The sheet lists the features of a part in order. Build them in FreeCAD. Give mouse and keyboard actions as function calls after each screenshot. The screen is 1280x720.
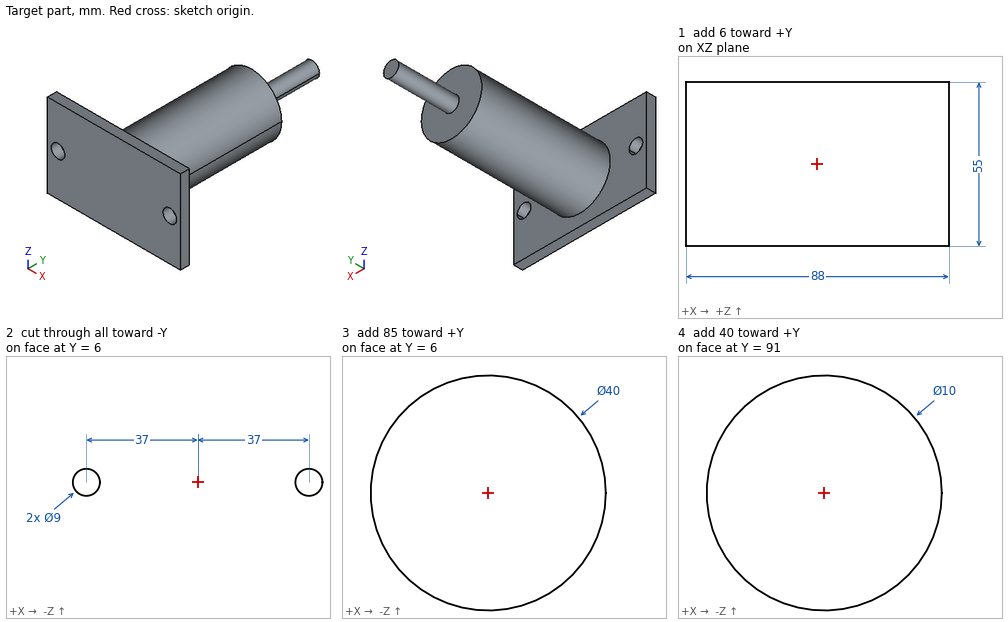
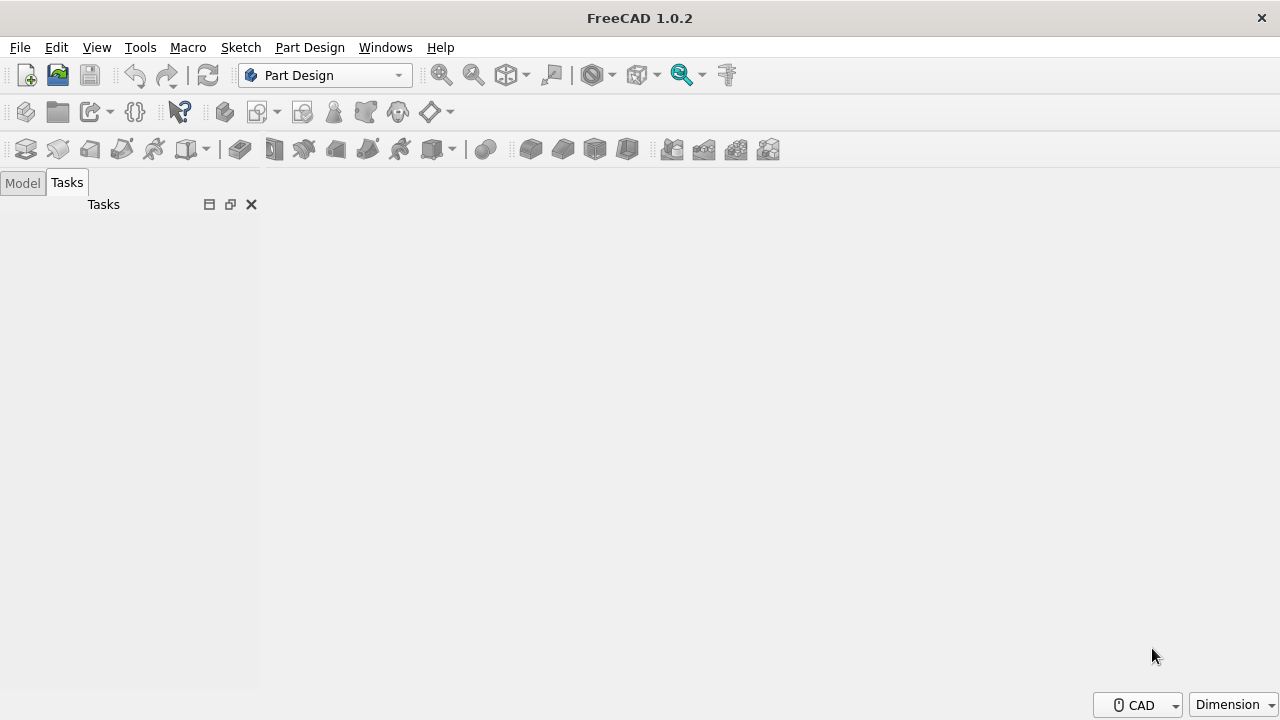
key(ctrl+n)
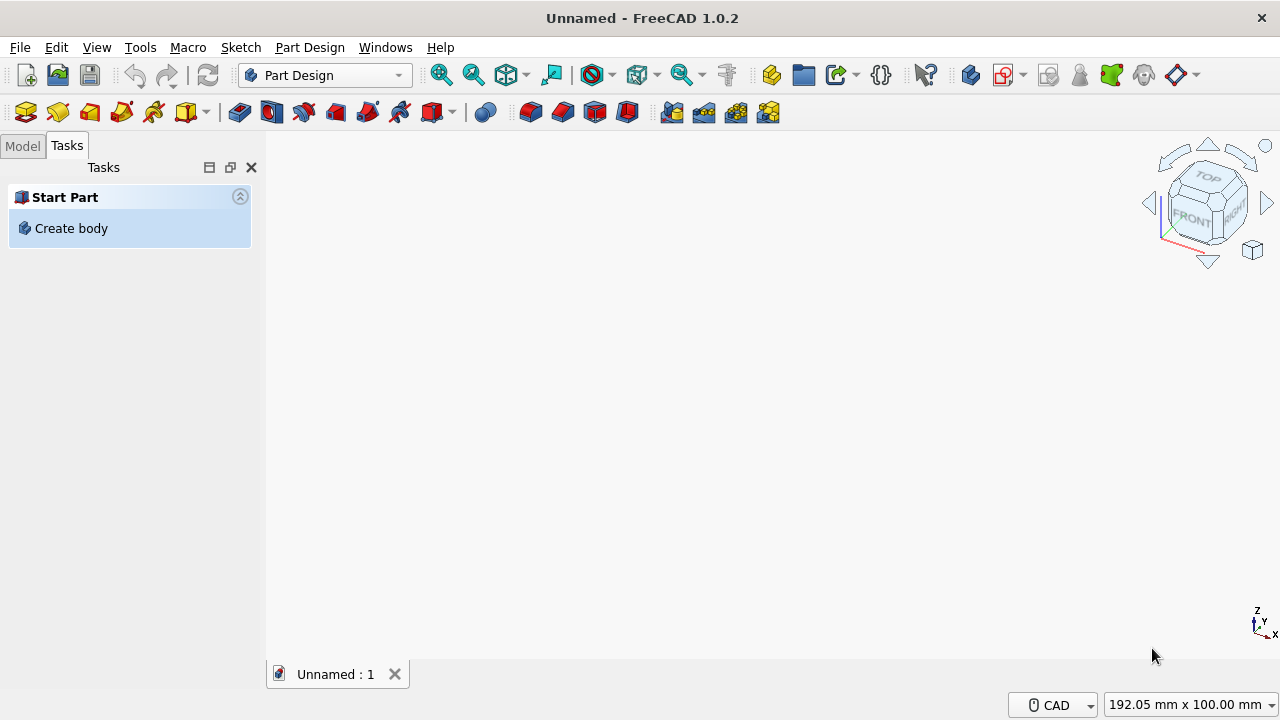
click(1004, 76)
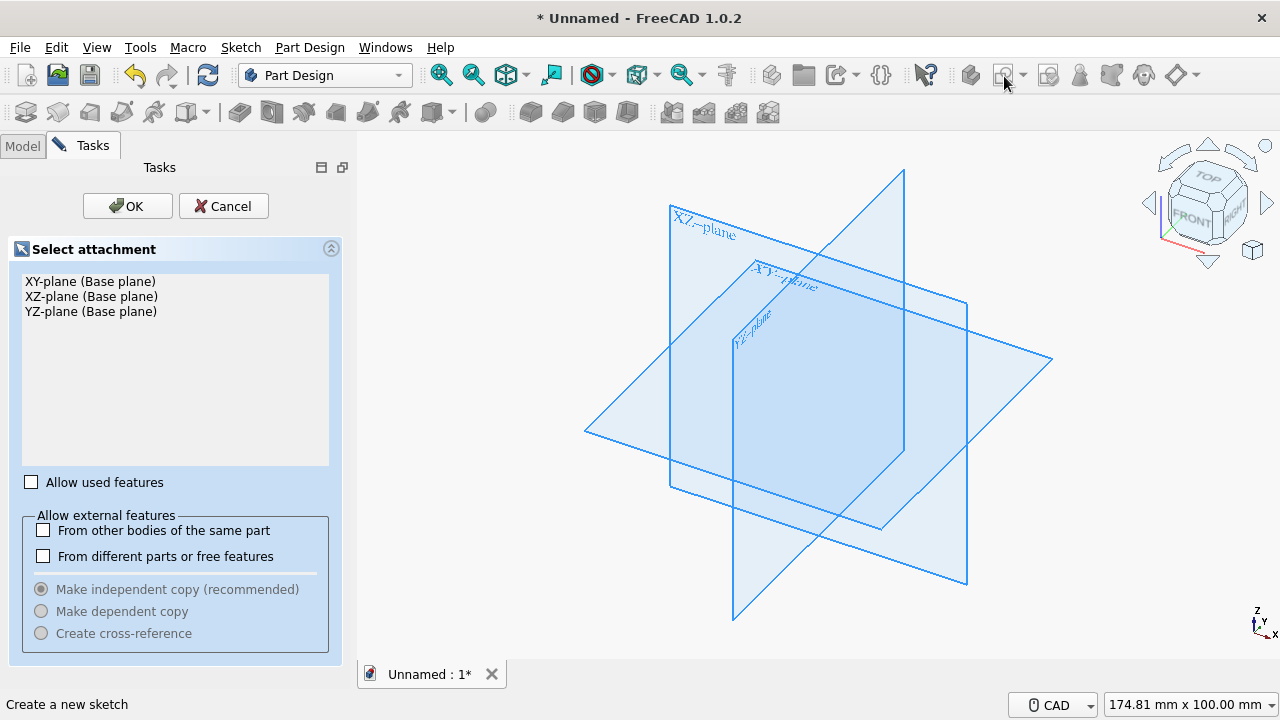
click(82, 296)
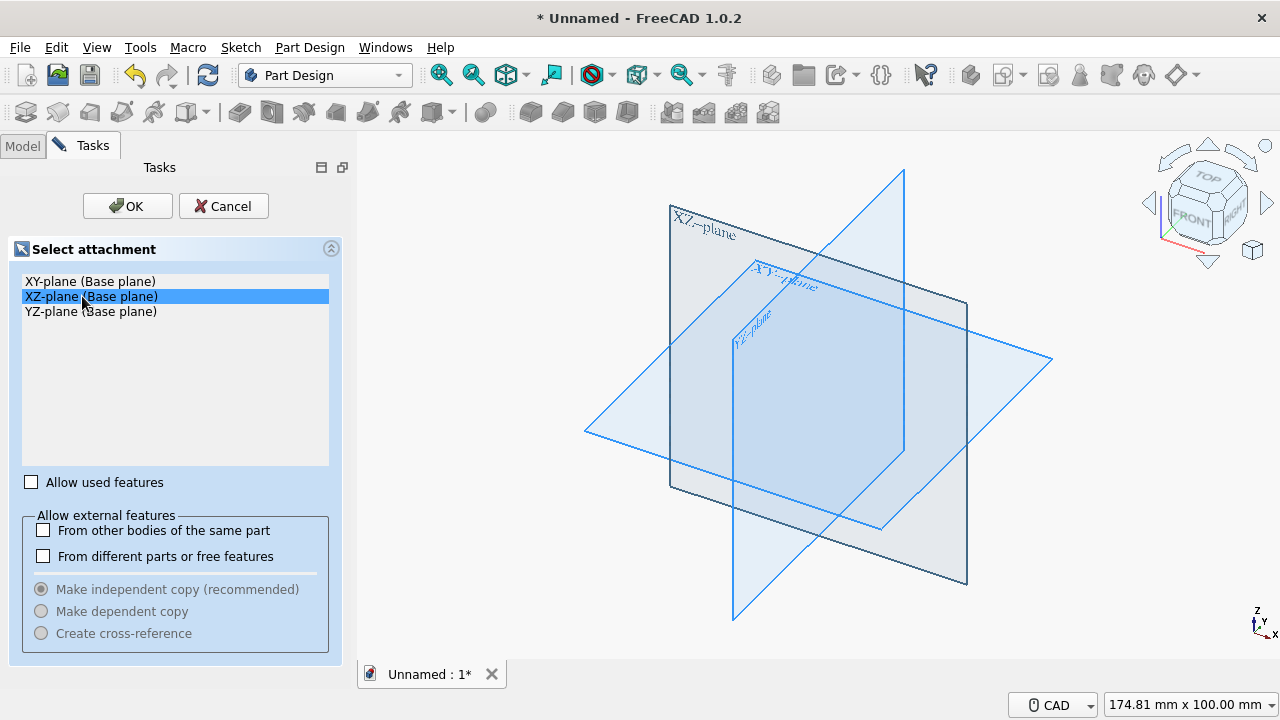
click(128, 206)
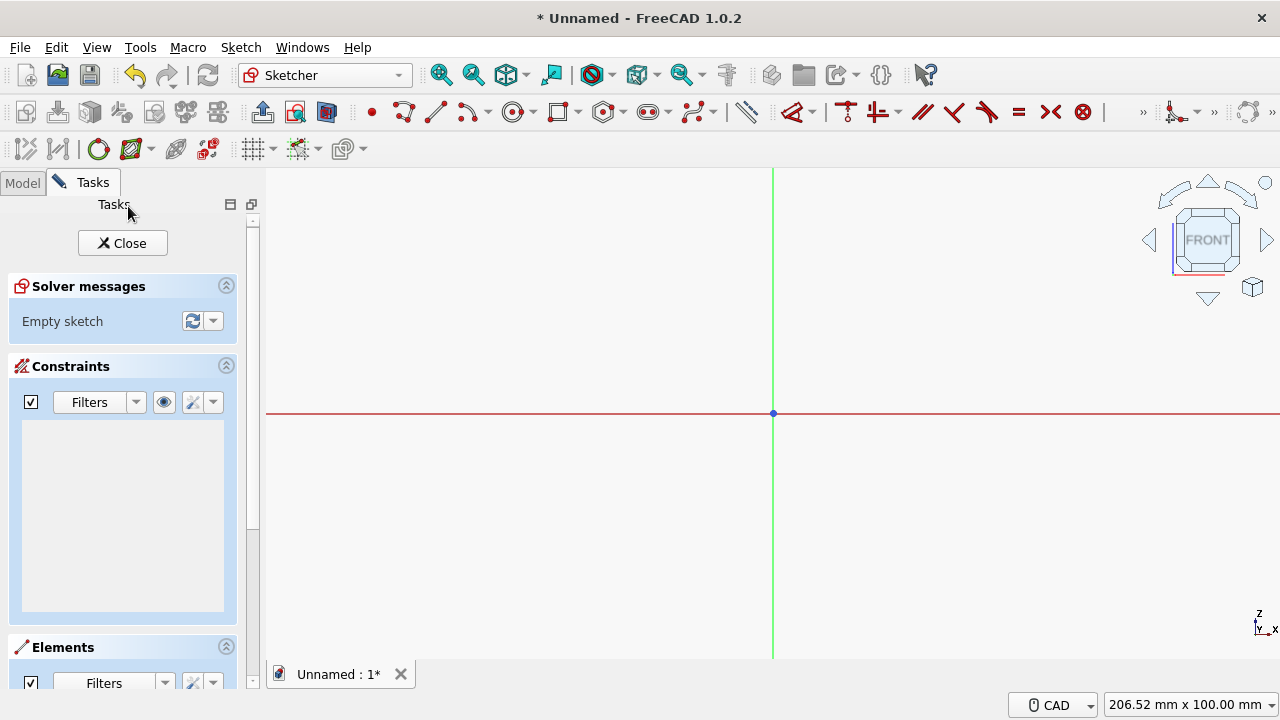
key(g)
key(v)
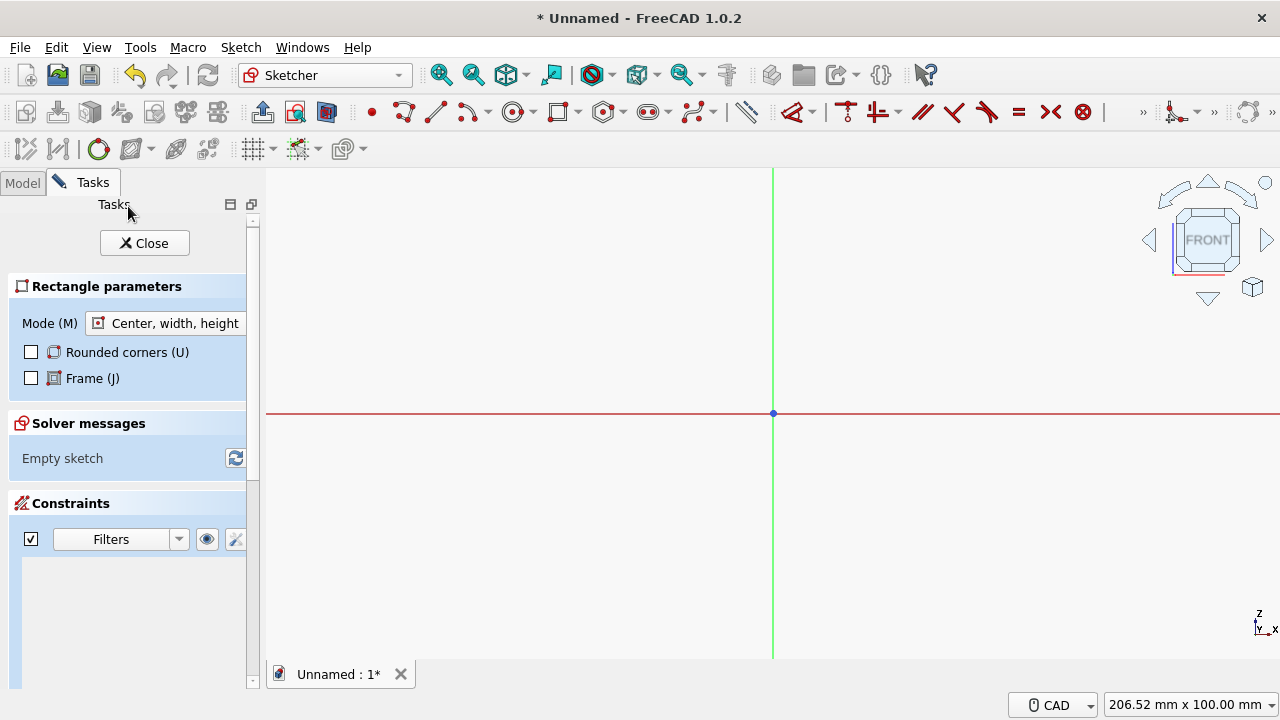
click(773, 414)
click(989, 278)
key(Escape)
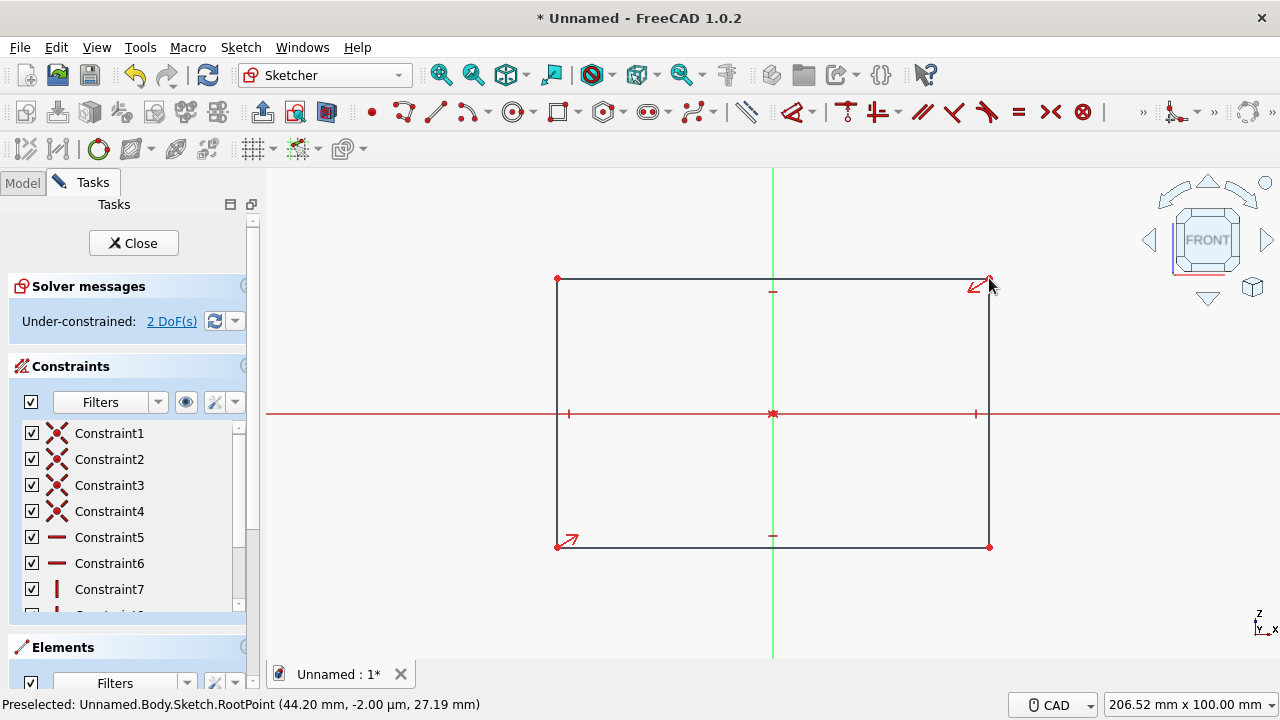
click(687, 548)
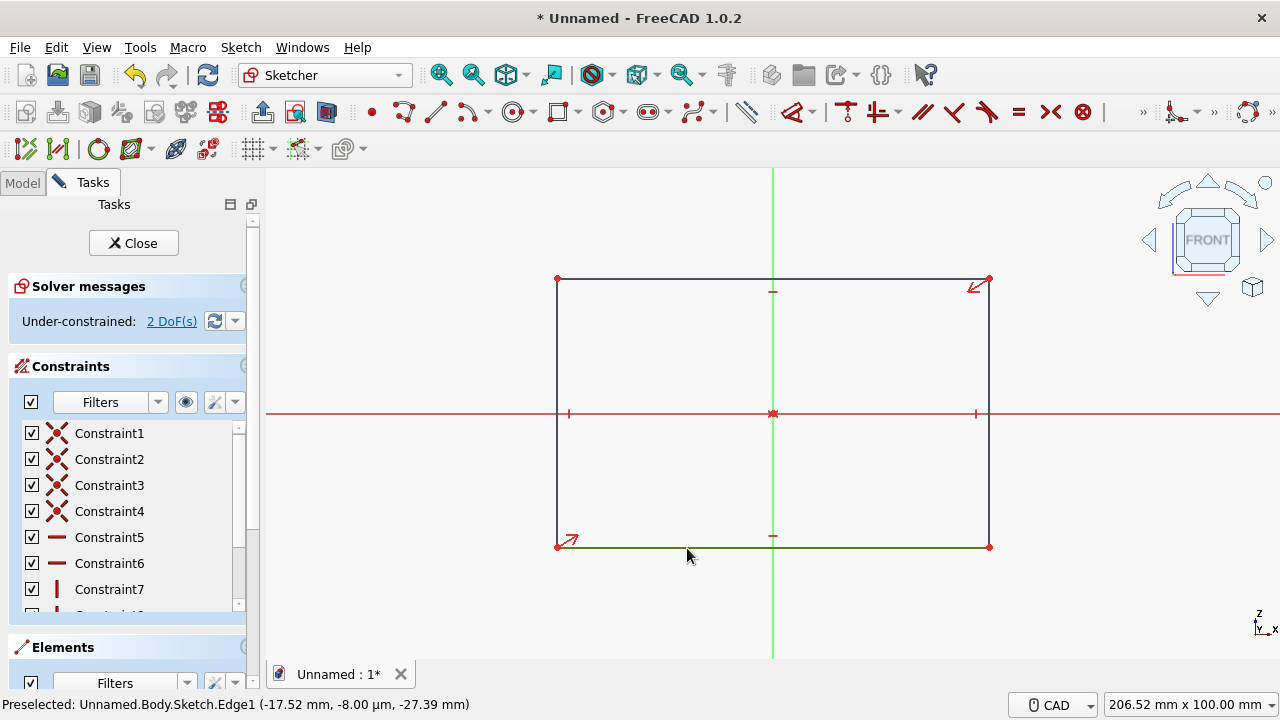
key(l)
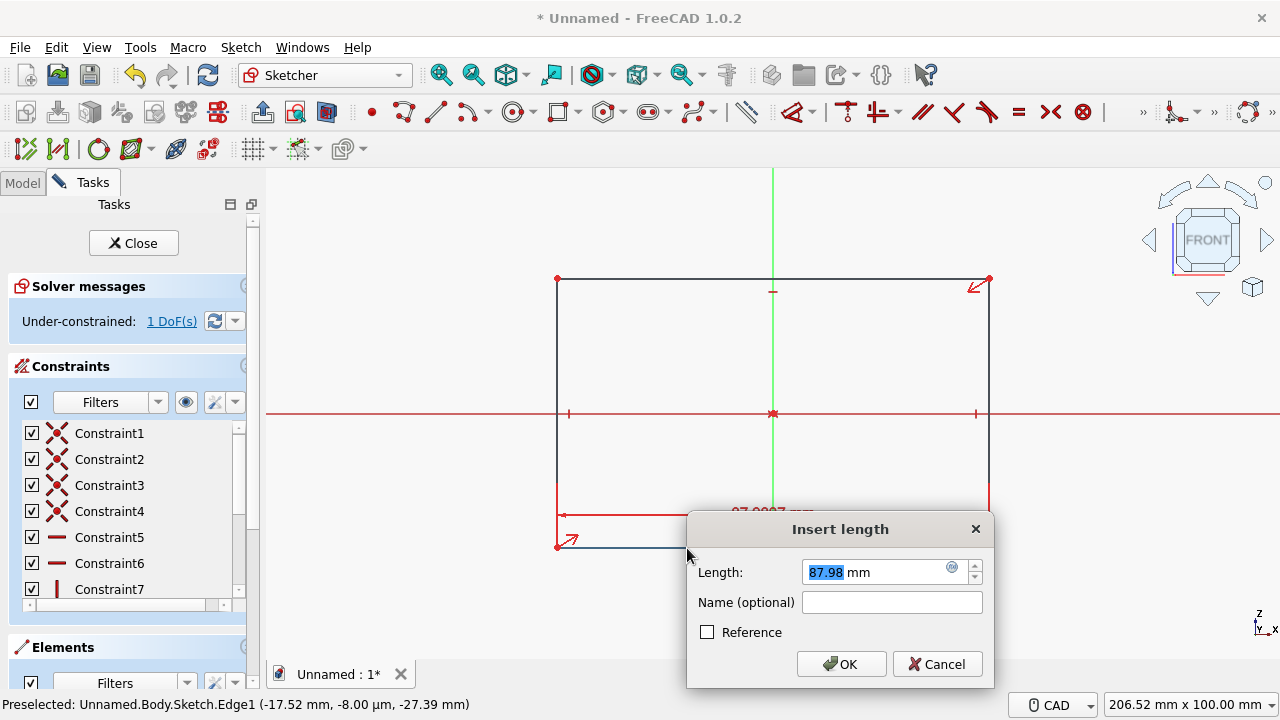
text(88)
key(Return)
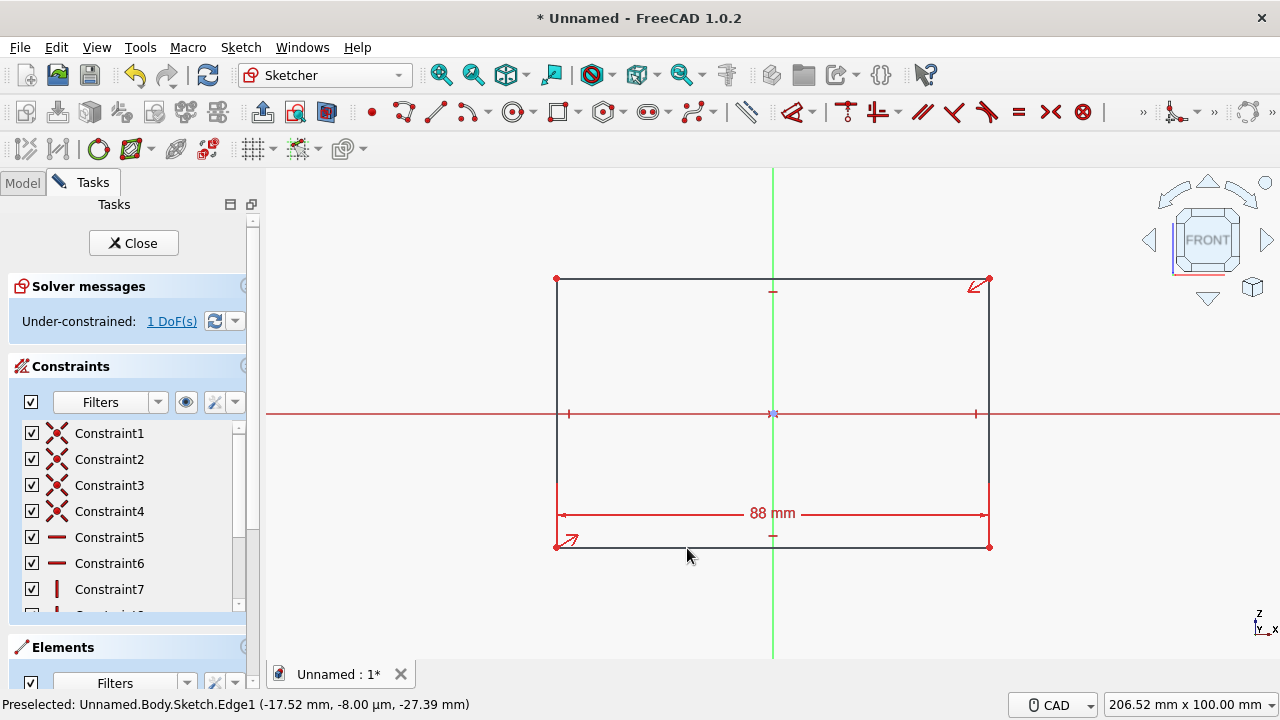
click(989, 467)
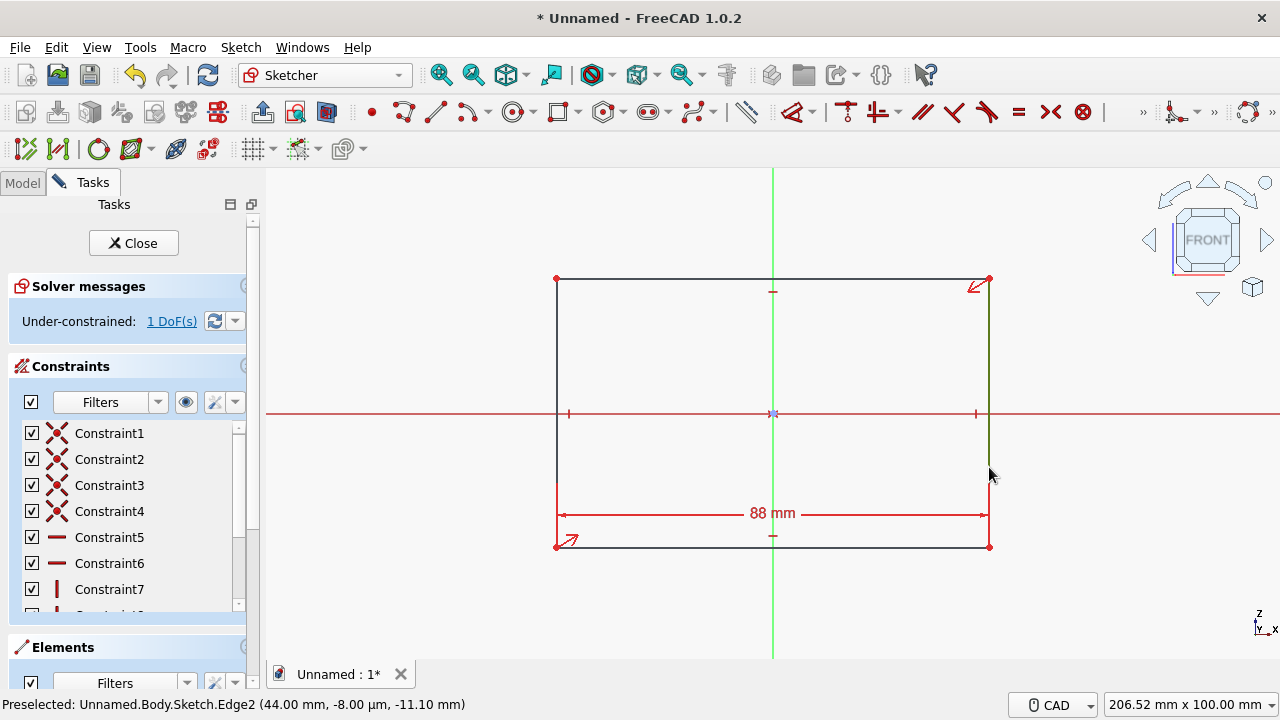
key(i)